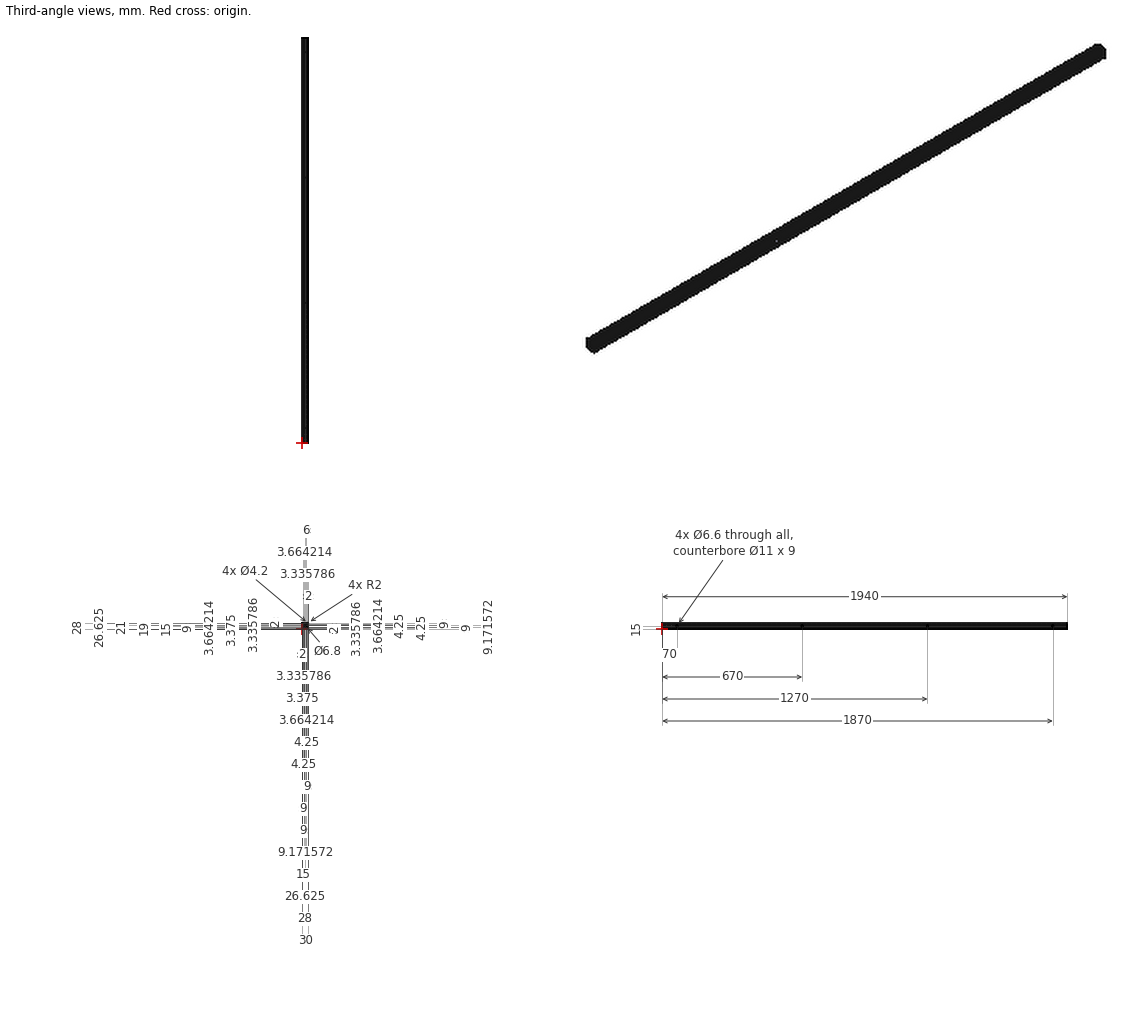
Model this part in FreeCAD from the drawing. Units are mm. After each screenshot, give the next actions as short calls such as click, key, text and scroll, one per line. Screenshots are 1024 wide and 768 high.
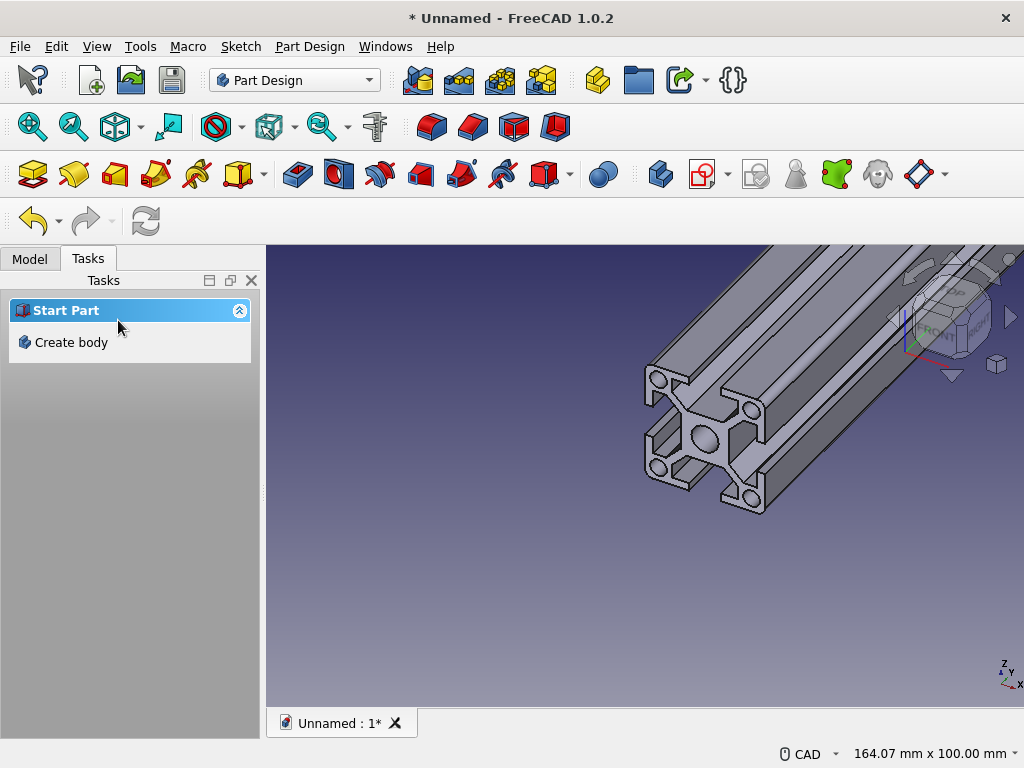
key(v)
key(f)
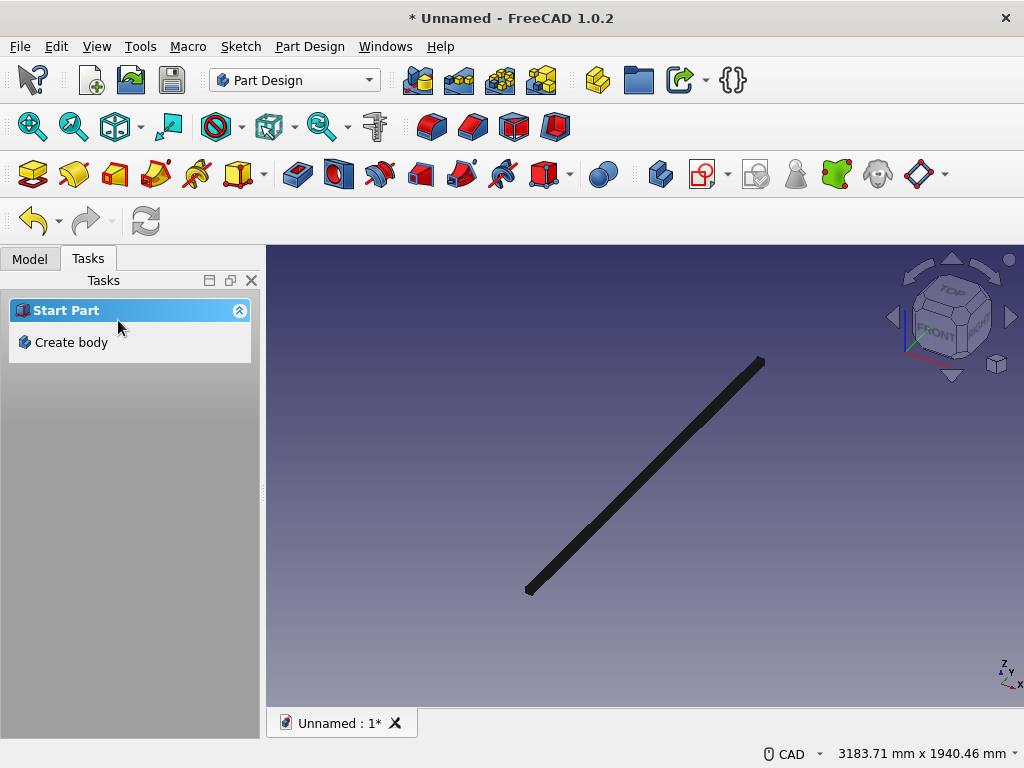
key(6)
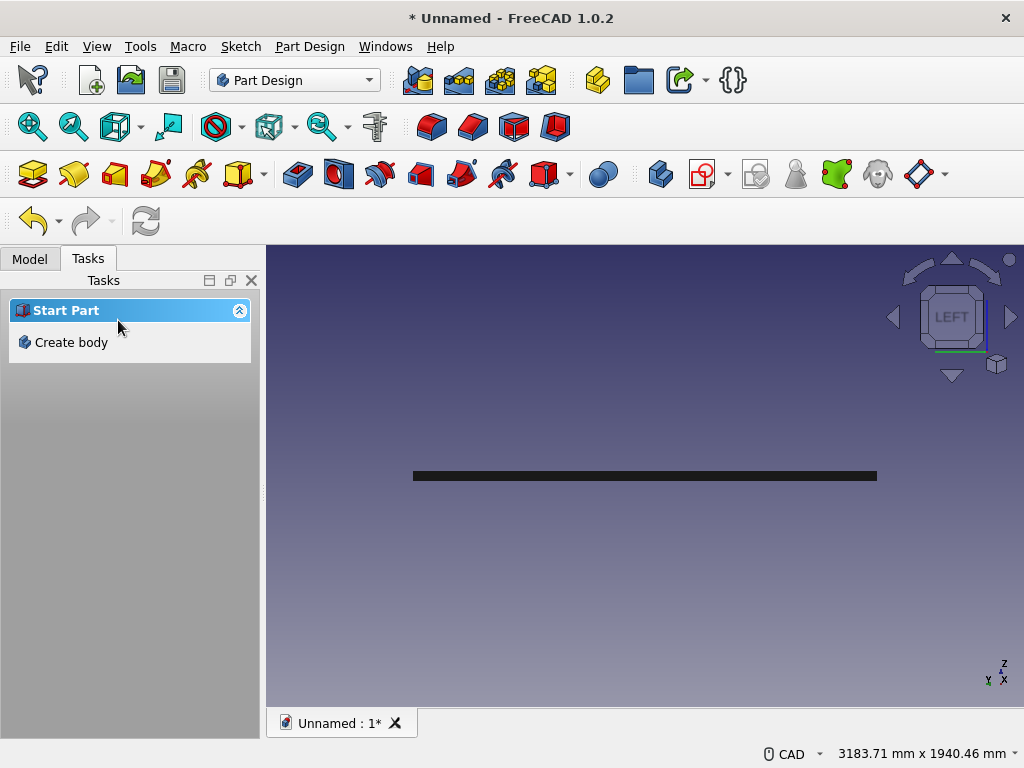
scroll(447, 473, up, 13)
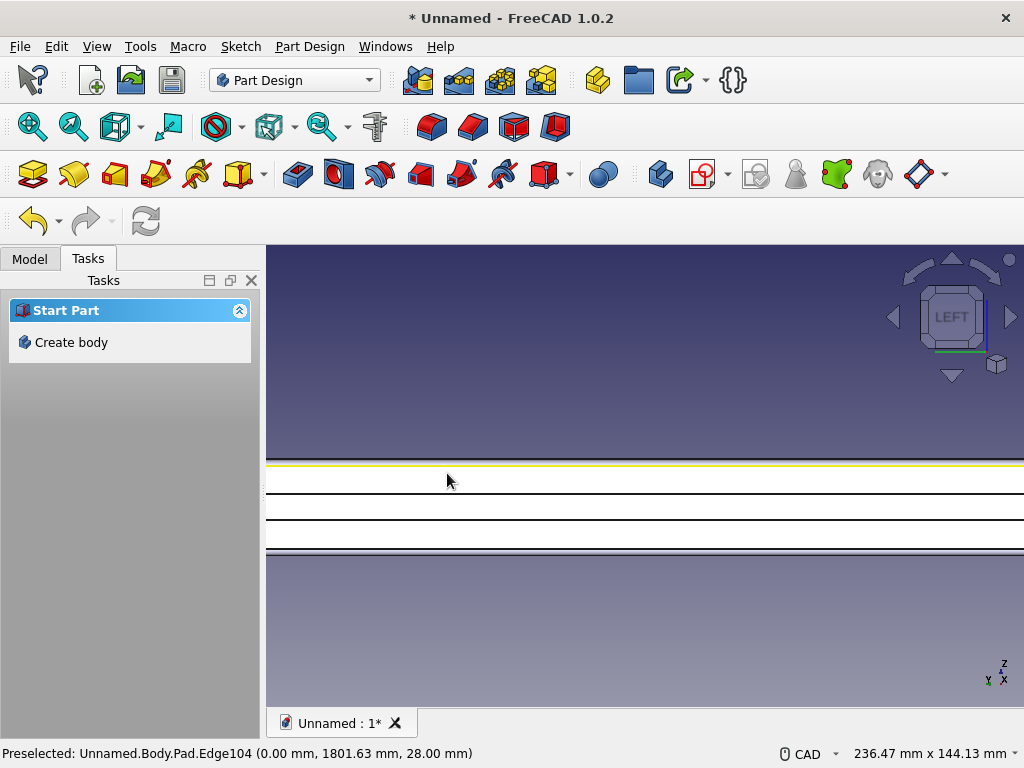
click(445, 479)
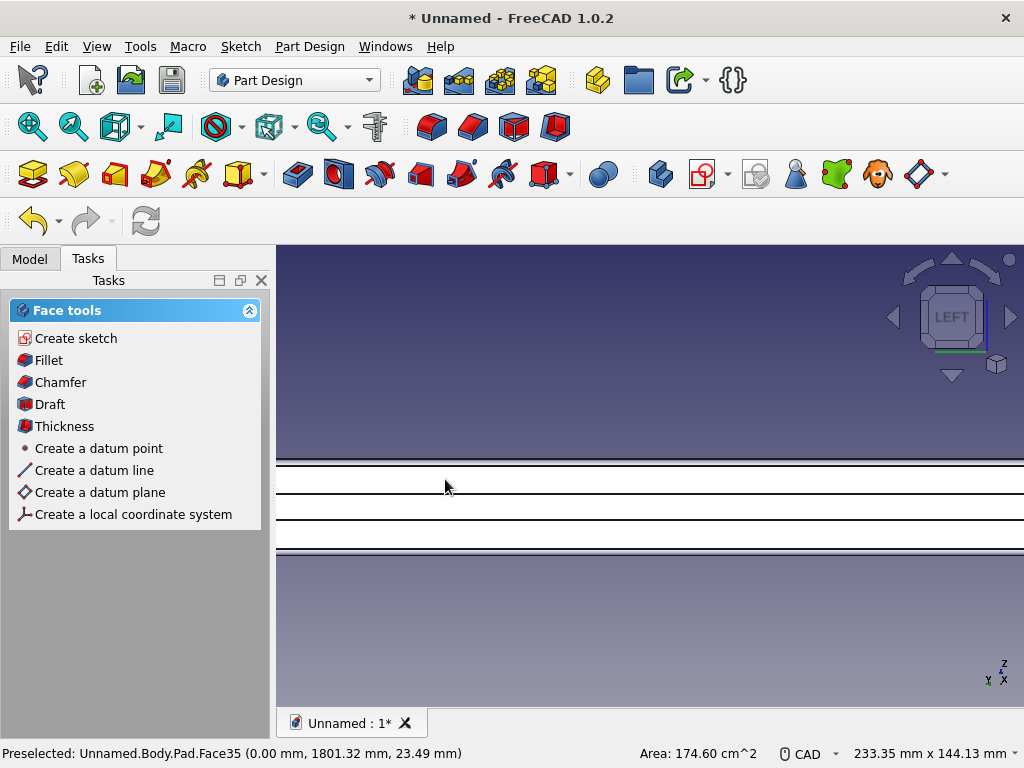
click(702, 174)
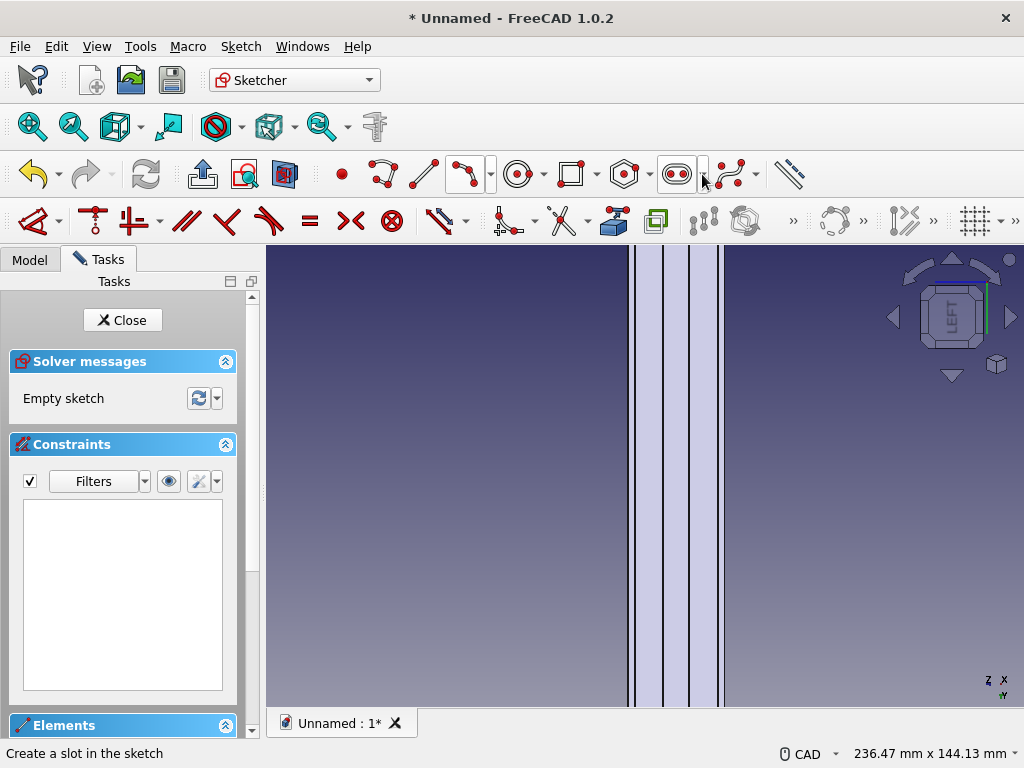
scroll(570, 611, down, 15)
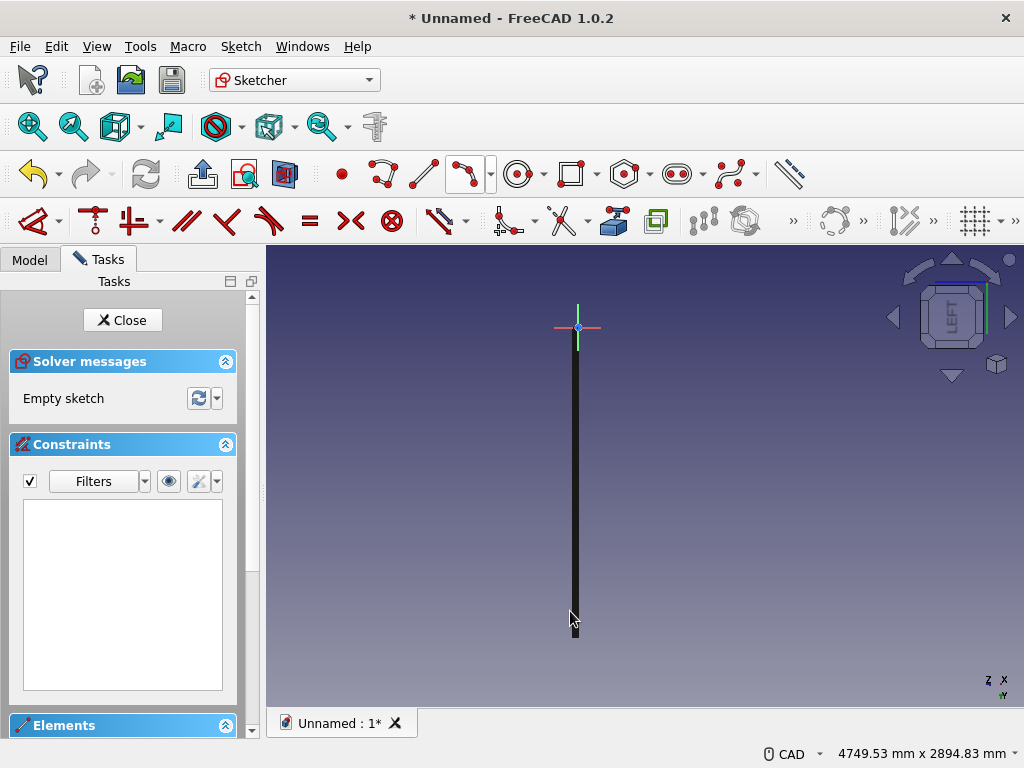
key(g)
key(c)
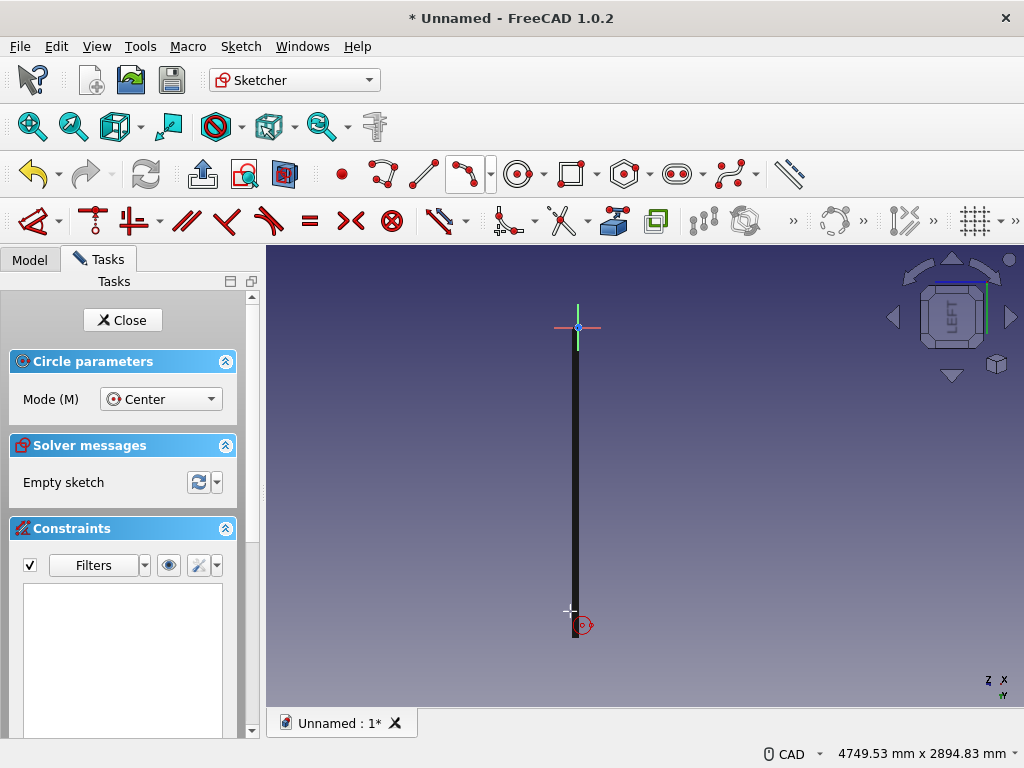
scroll(576, 339, up, 19)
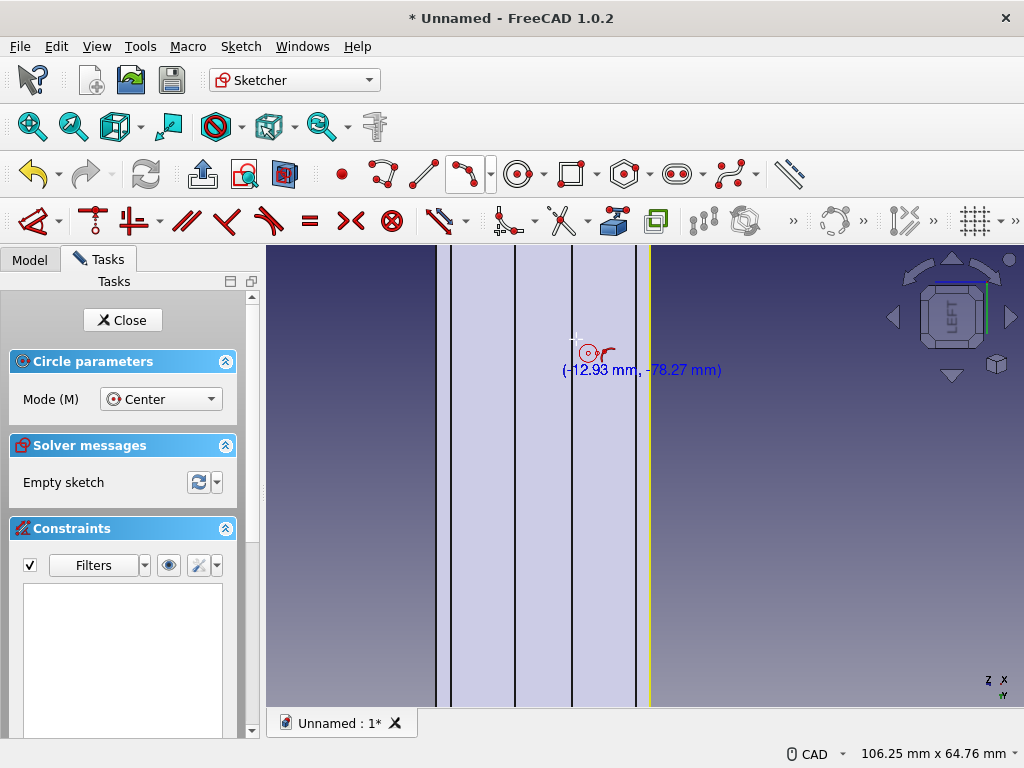
scroll(576, 476, down, 15)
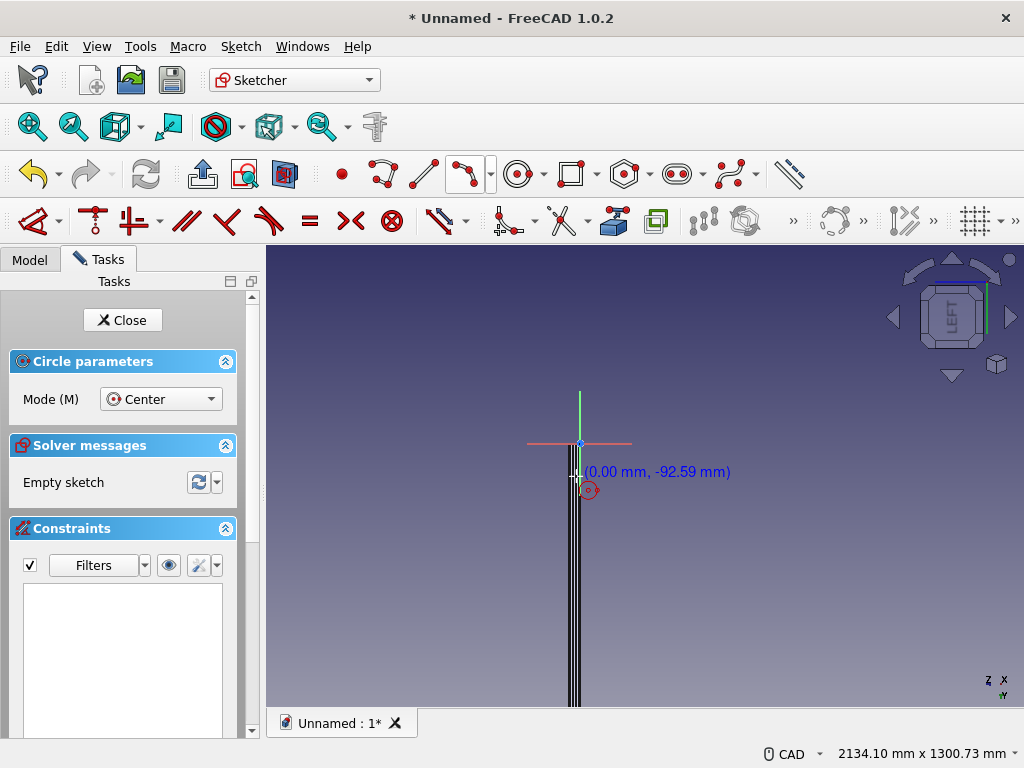
scroll(576, 273, down, 4)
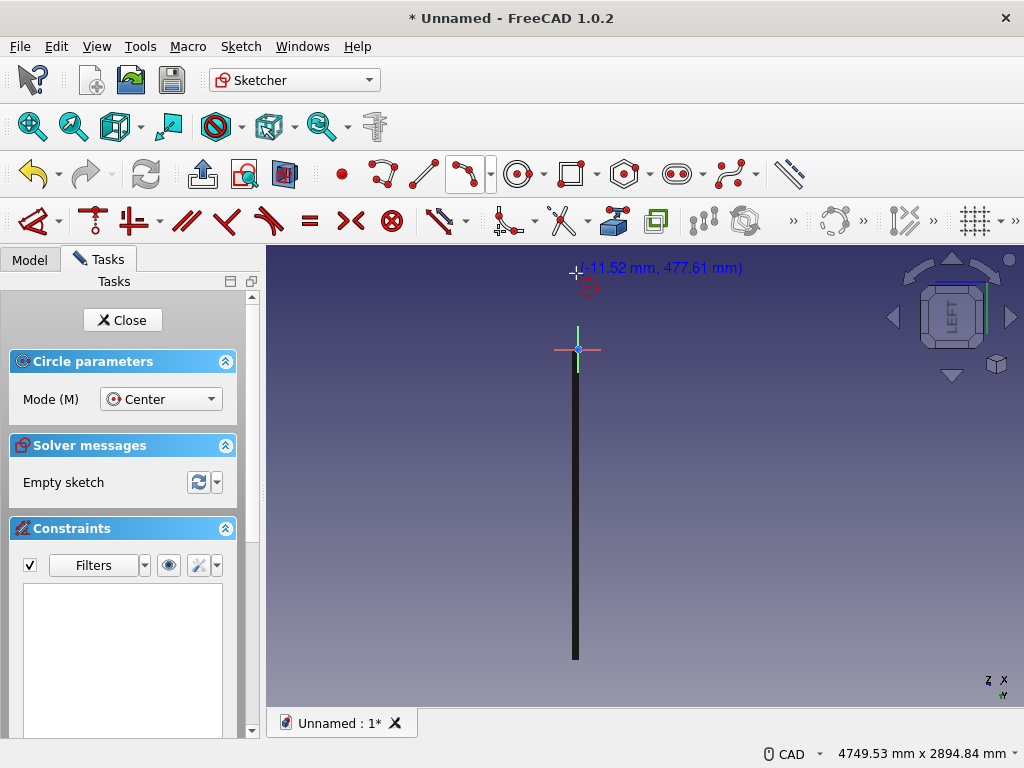
scroll(576, 361, up, 10)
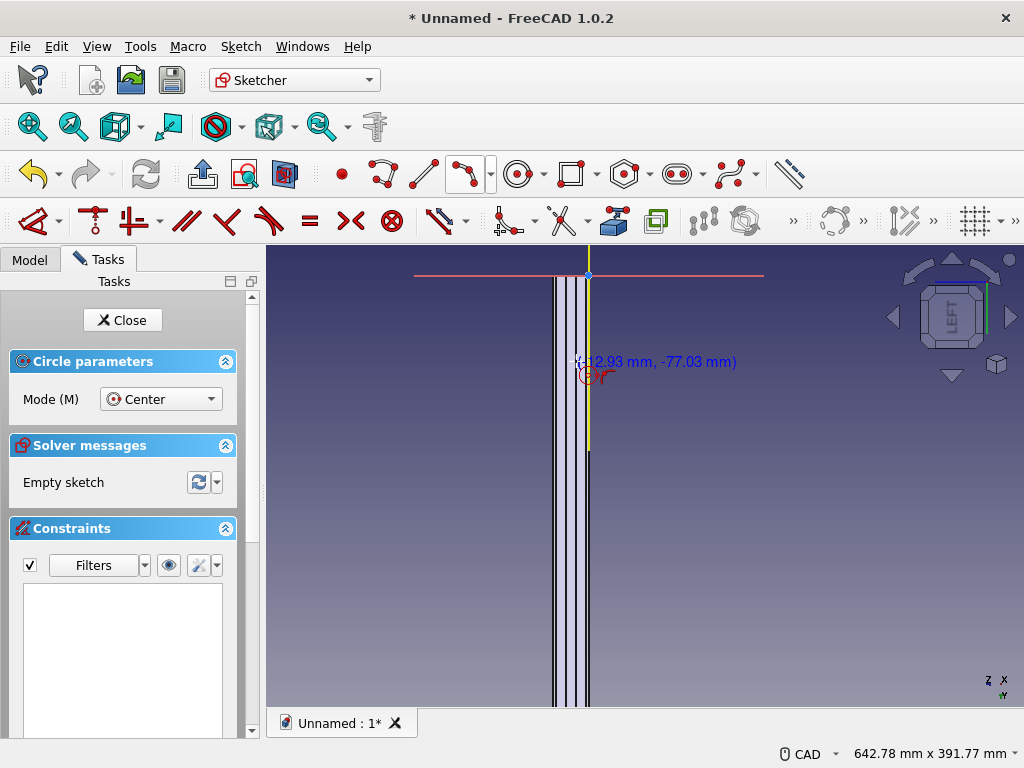
click(571, 358)